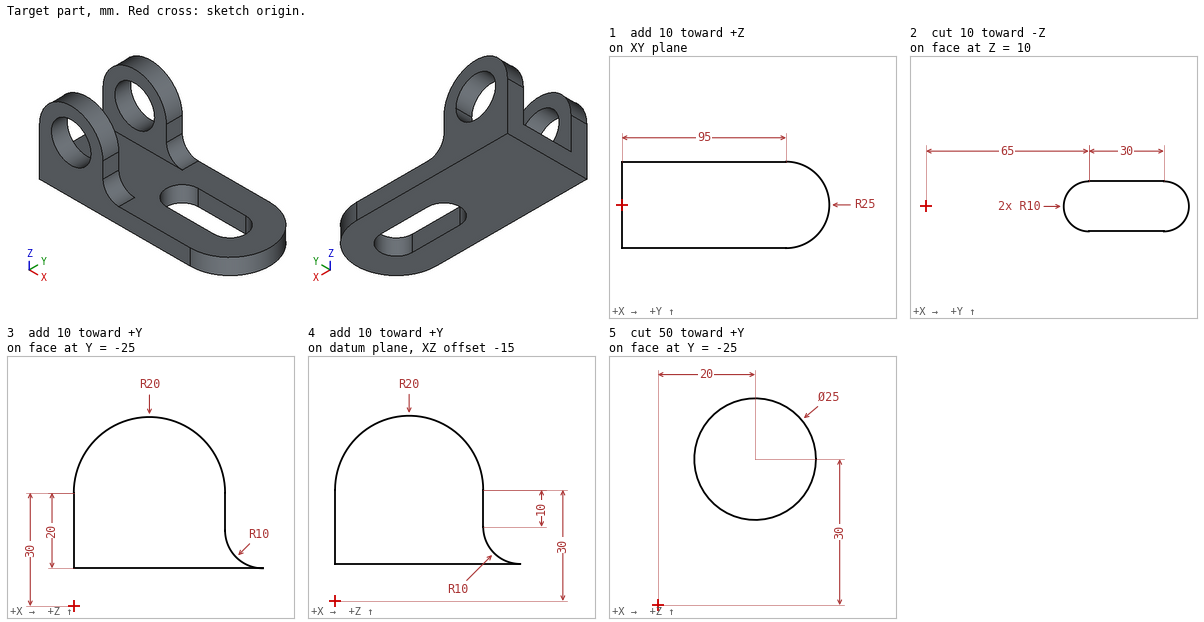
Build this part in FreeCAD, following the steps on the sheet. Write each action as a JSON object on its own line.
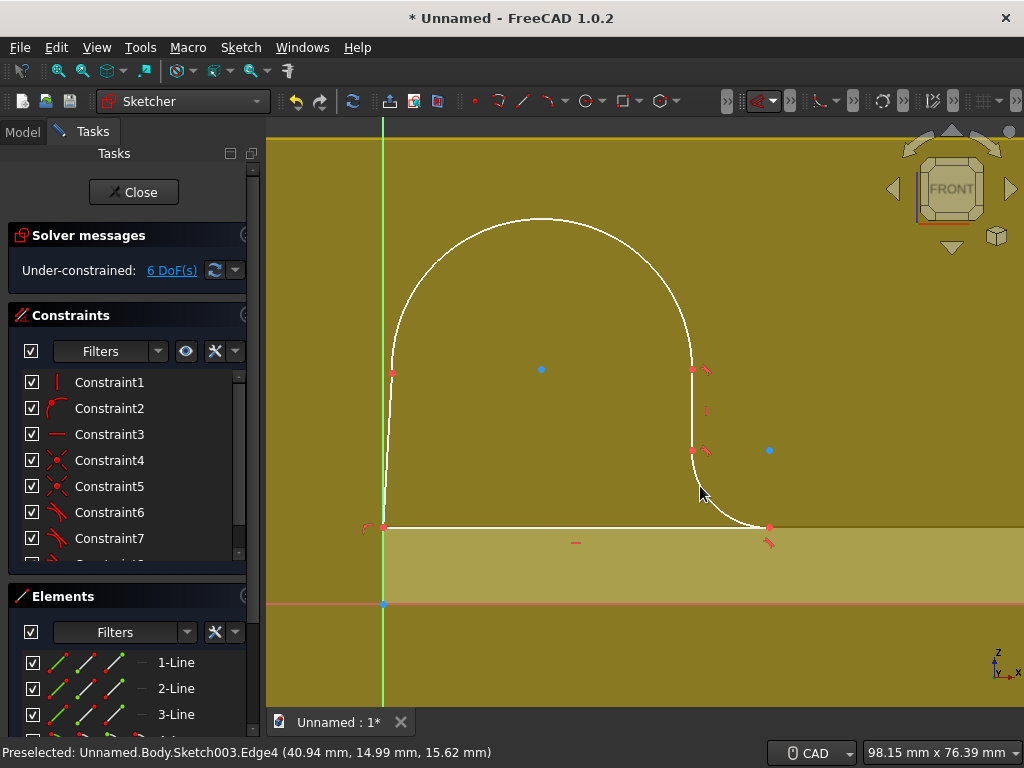
{"action": "left_click", "coordinate": [386, 482]}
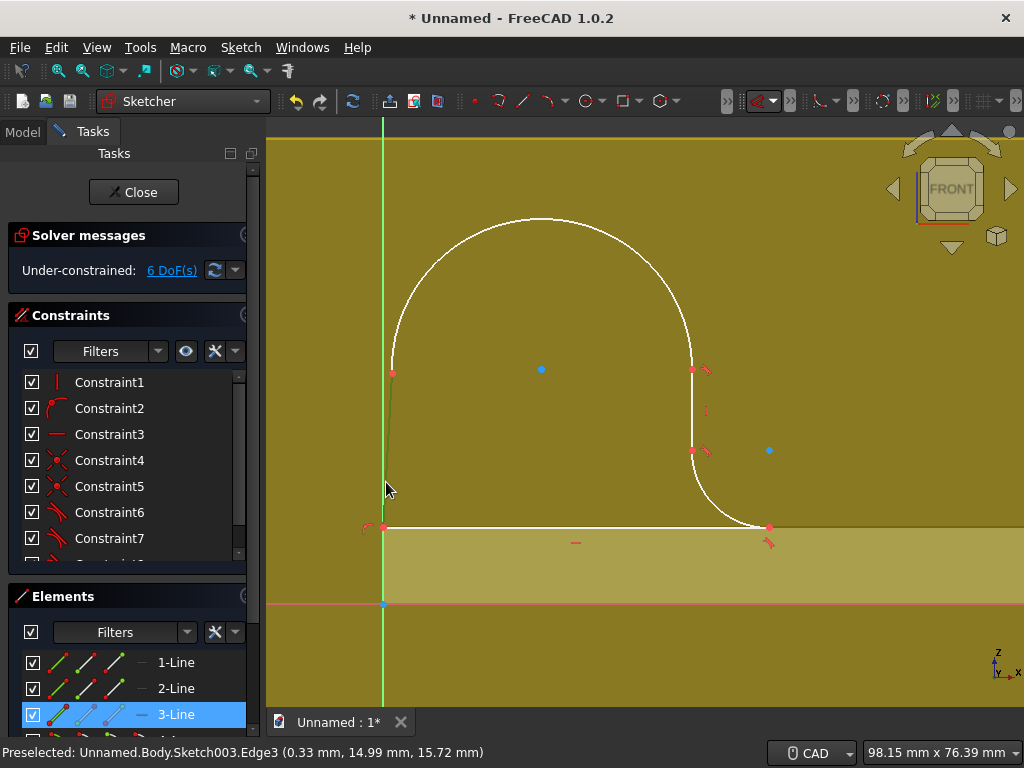
{"action": "left_click", "coordinate": [629, 247]}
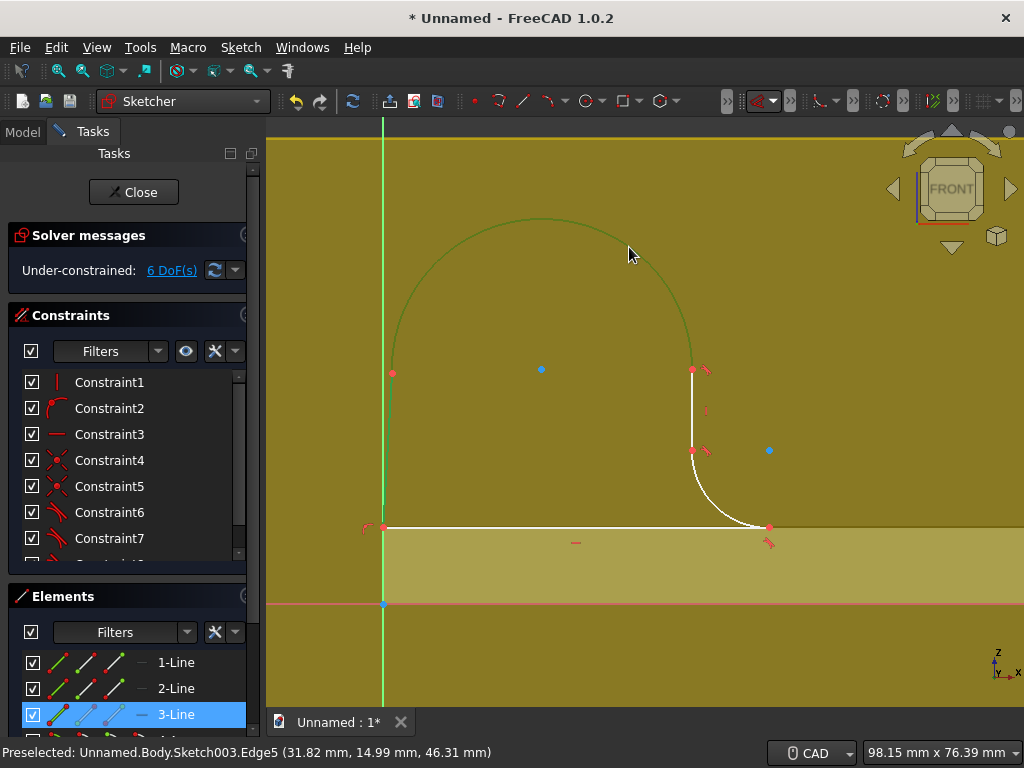
{"action": "key", "text": "t"}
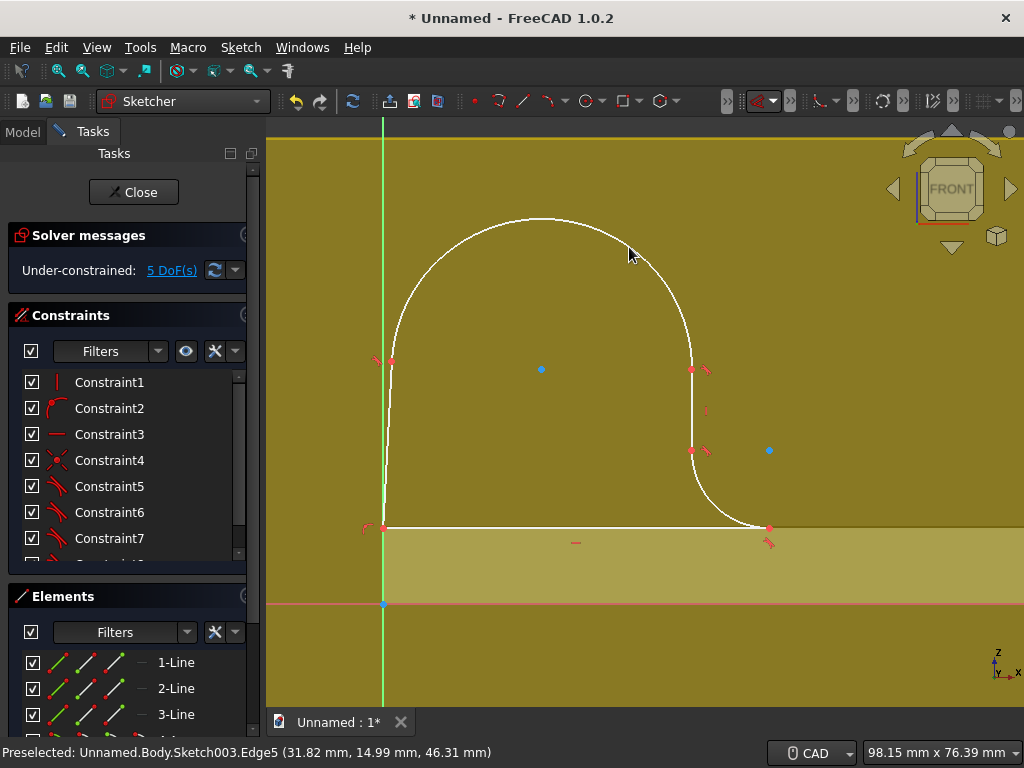
{"action": "left_click", "coordinate": [386, 478]}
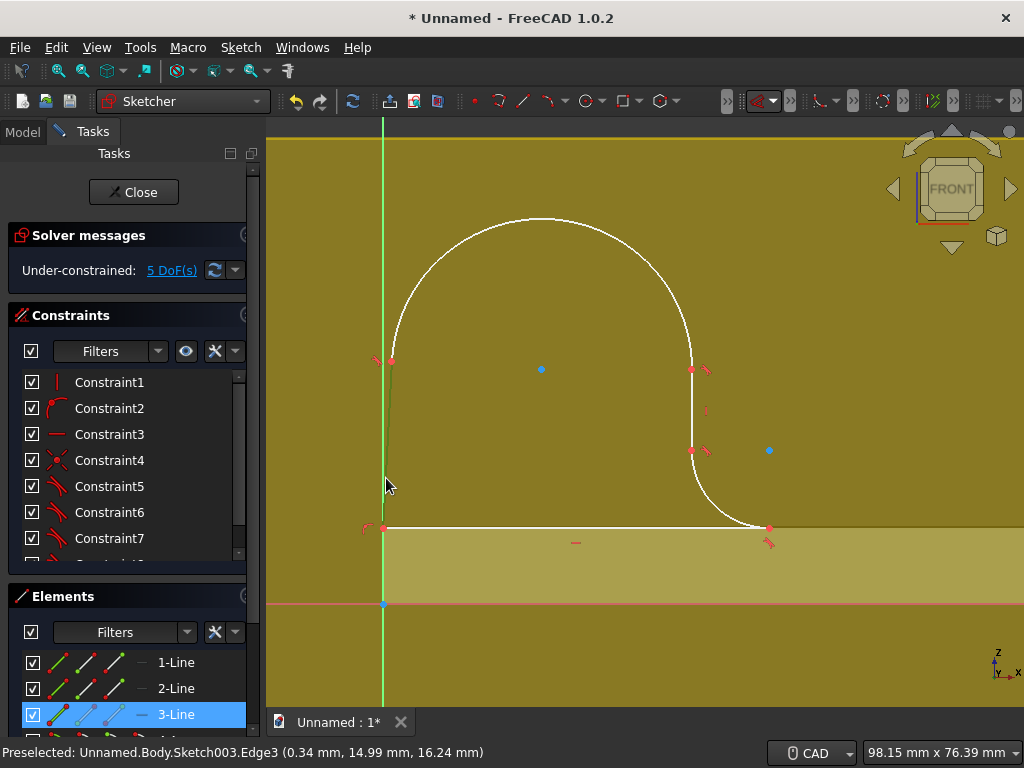
{"action": "key", "text": "v"}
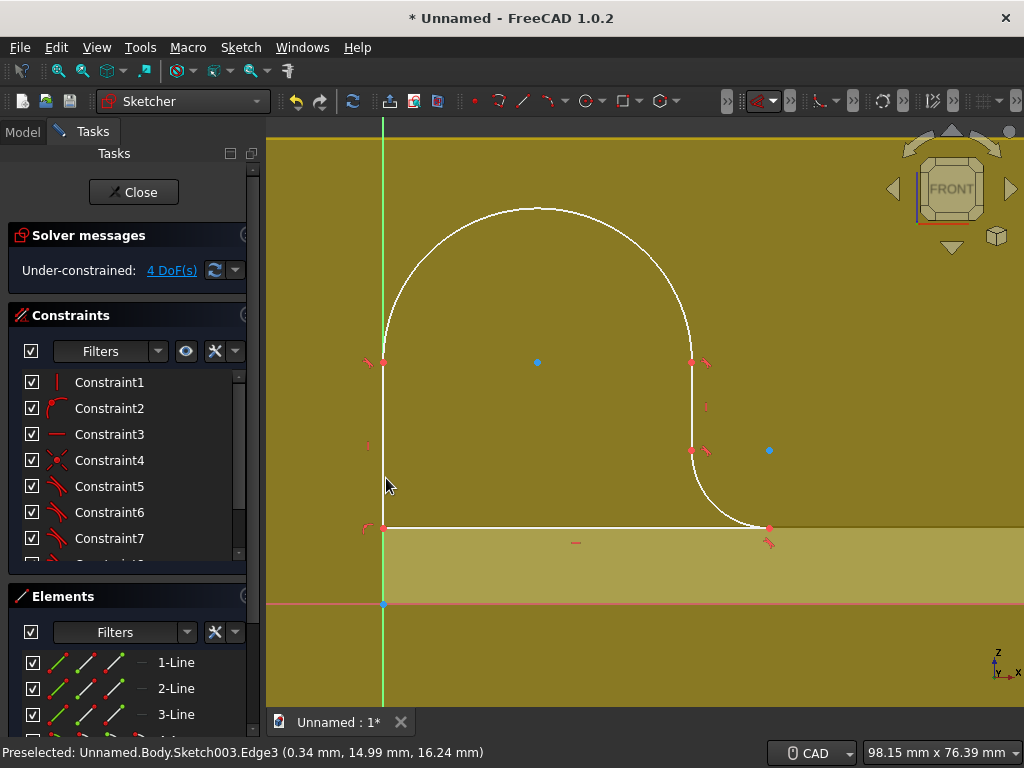
{"action": "left_click", "coordinate": [700, 486]}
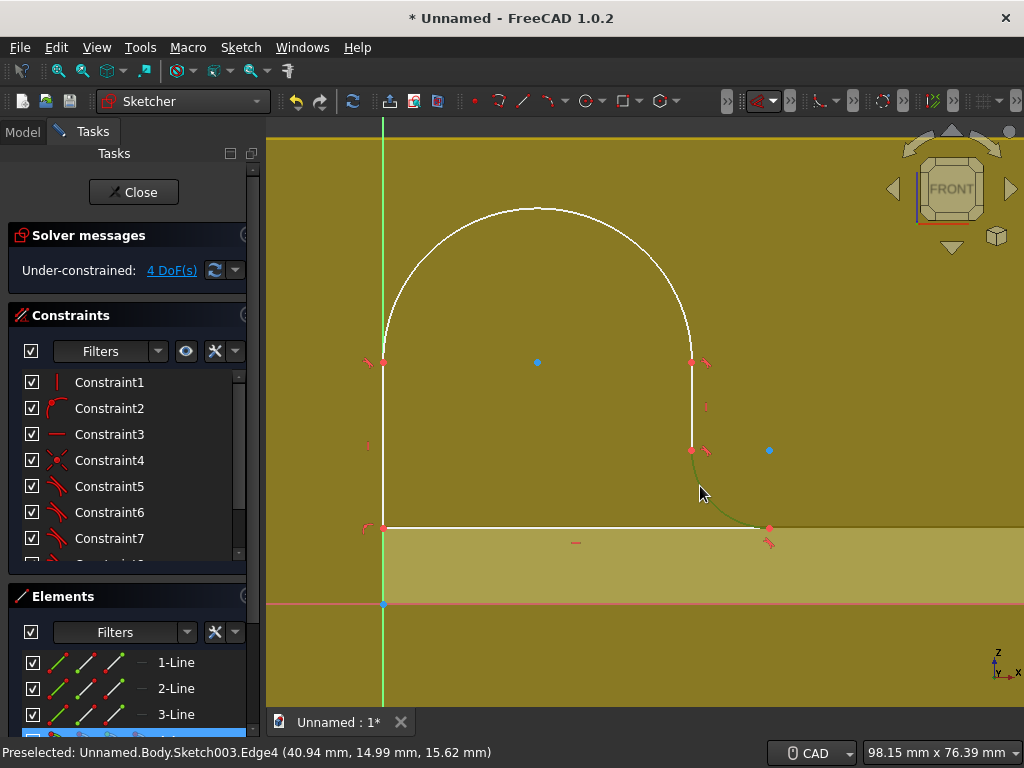
{"action": "left_click", "coordinate": [776, 102]}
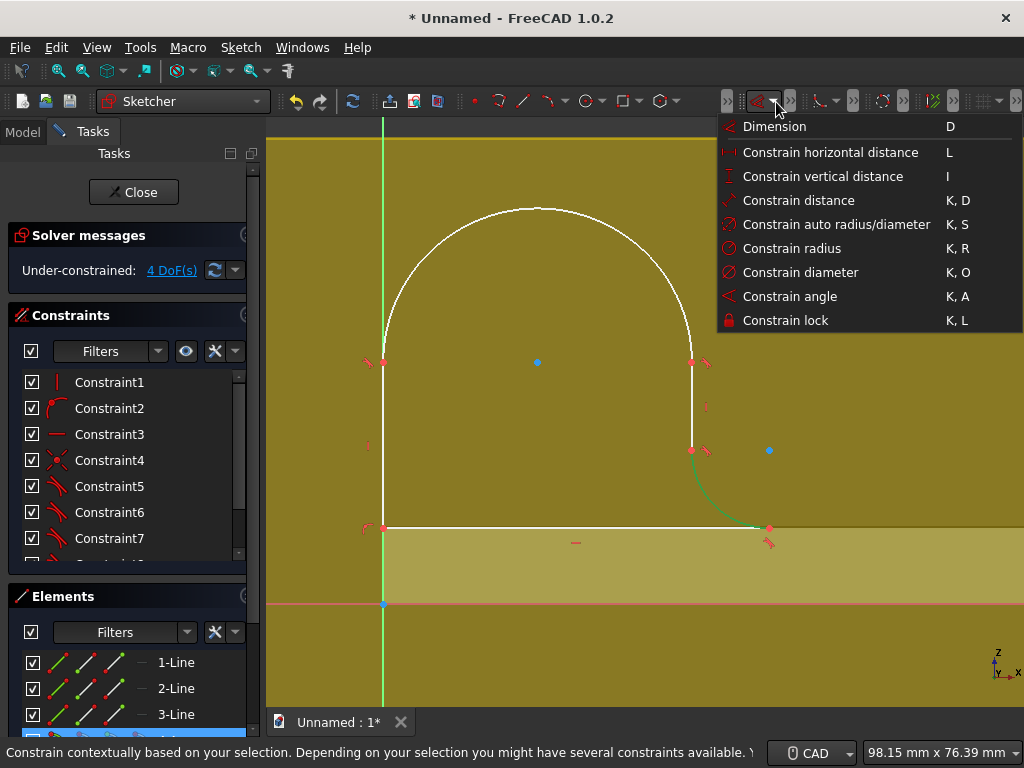
{"action": "left_click", "coordinate": [870, 248]}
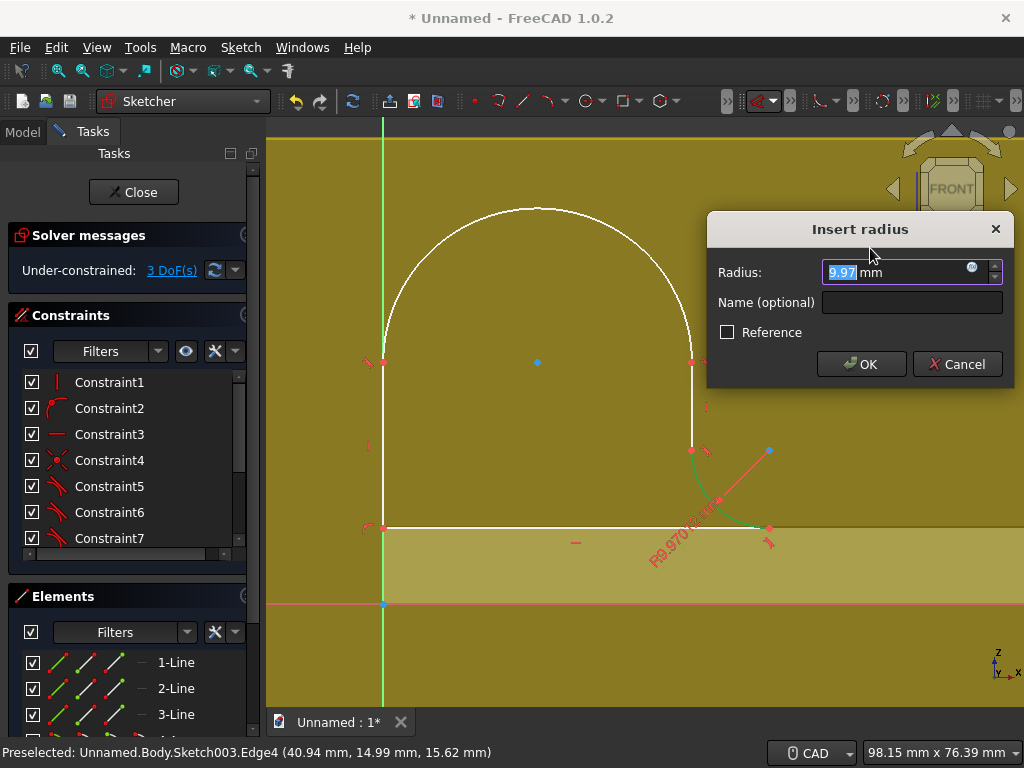
{"action": "type", "text": "10"}
{"action": "key", "text": "Return"}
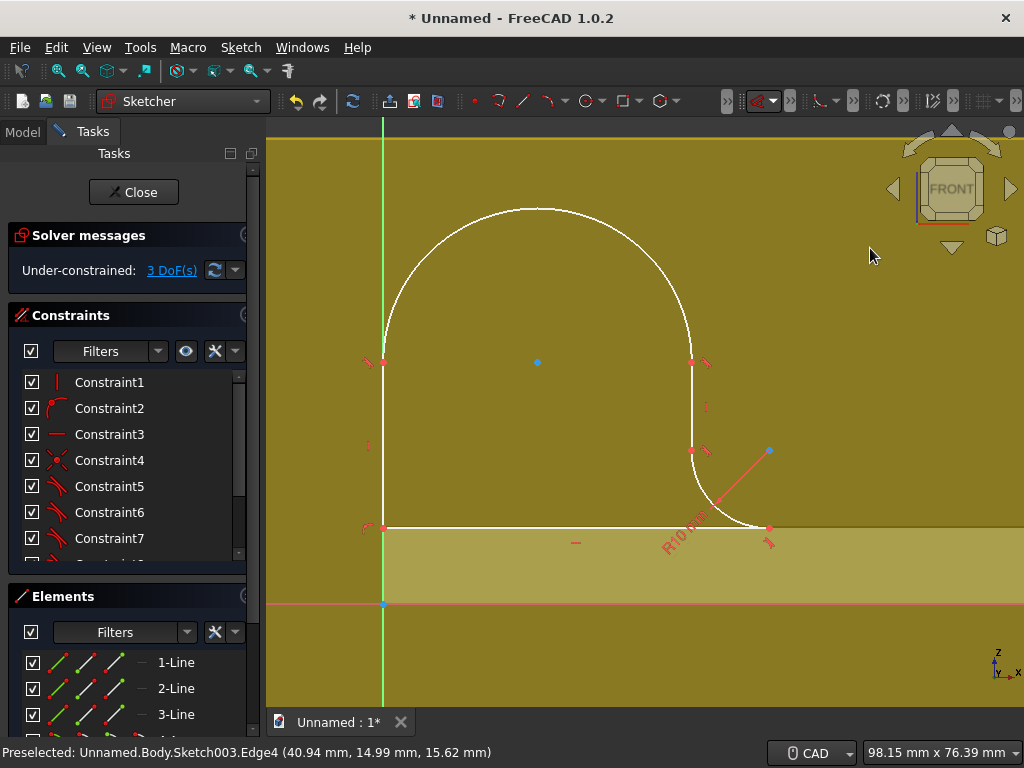
{"action": "left_click", "coordinate": [628, 238]}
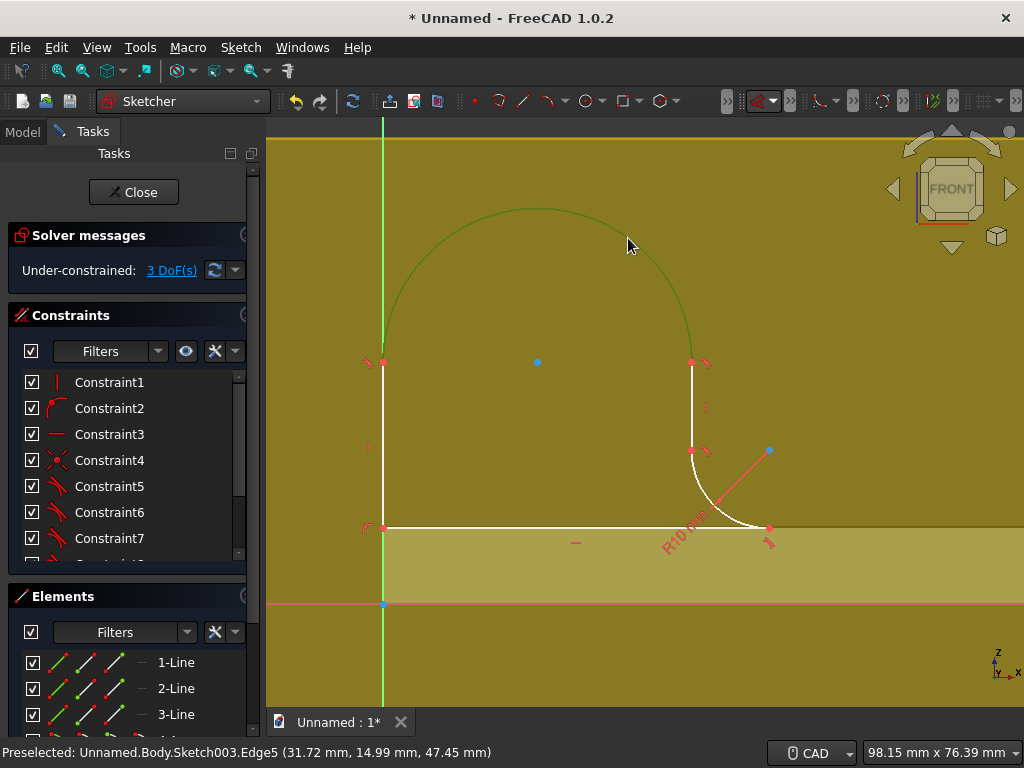
{"action": "left_click", "coordinate": [776, 102]}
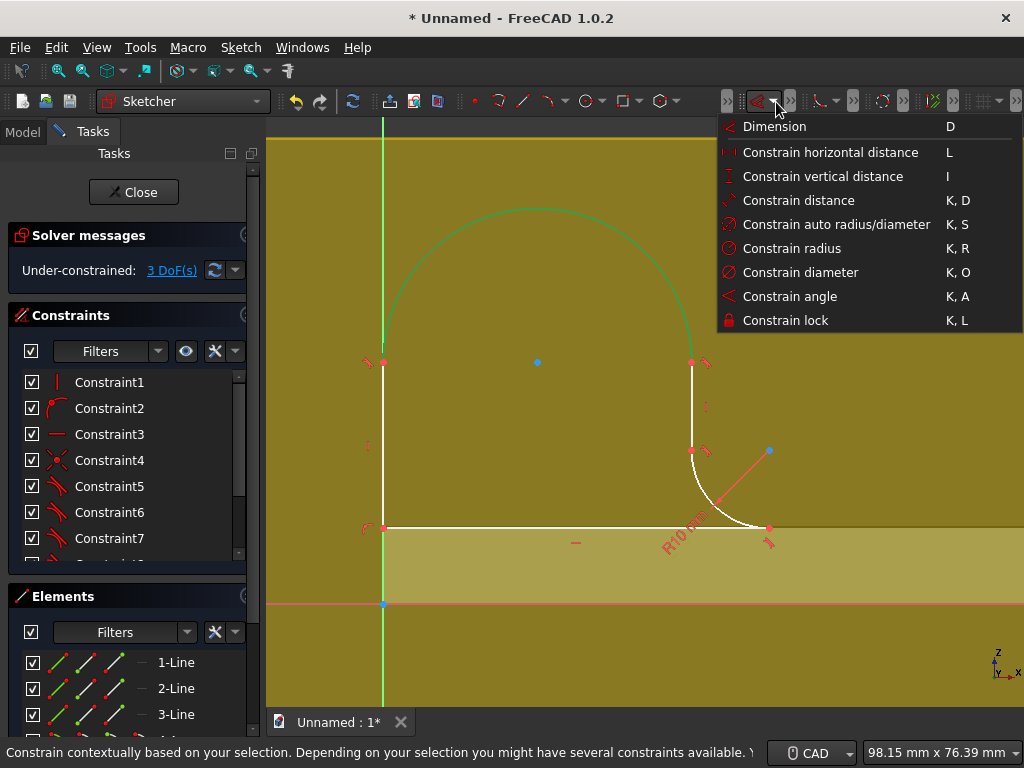
{"action": "left_click", "coordinate": [870, 248]}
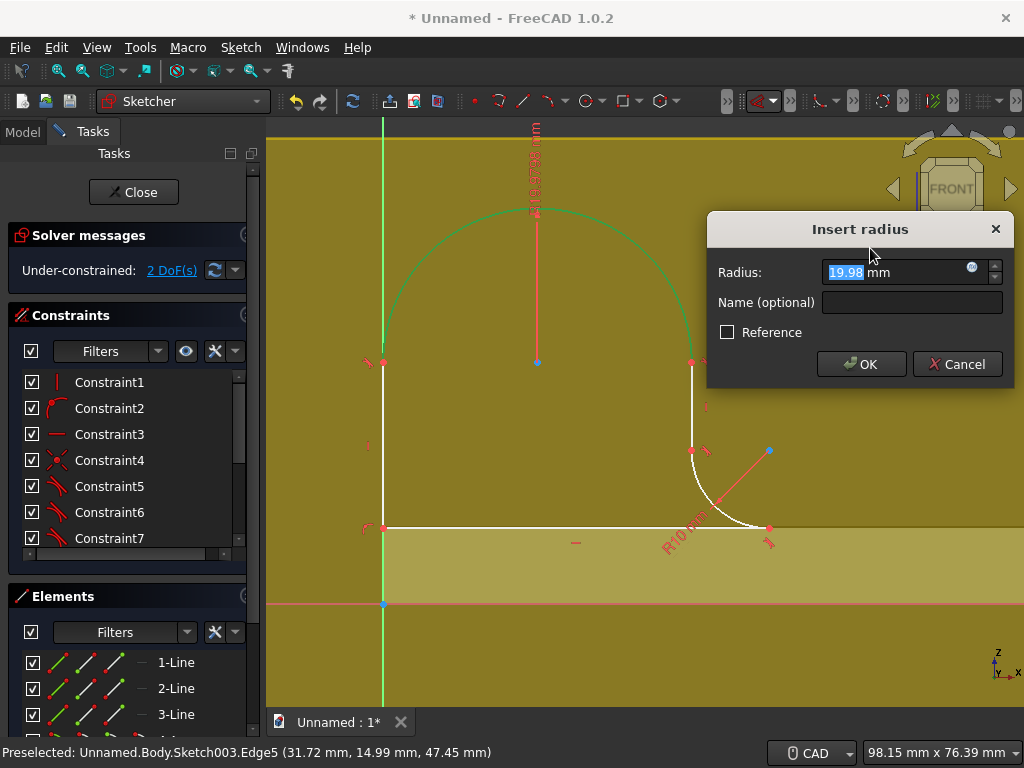
{"action": "type", "text": "20"}
{"action": "key", "text": "Return"}